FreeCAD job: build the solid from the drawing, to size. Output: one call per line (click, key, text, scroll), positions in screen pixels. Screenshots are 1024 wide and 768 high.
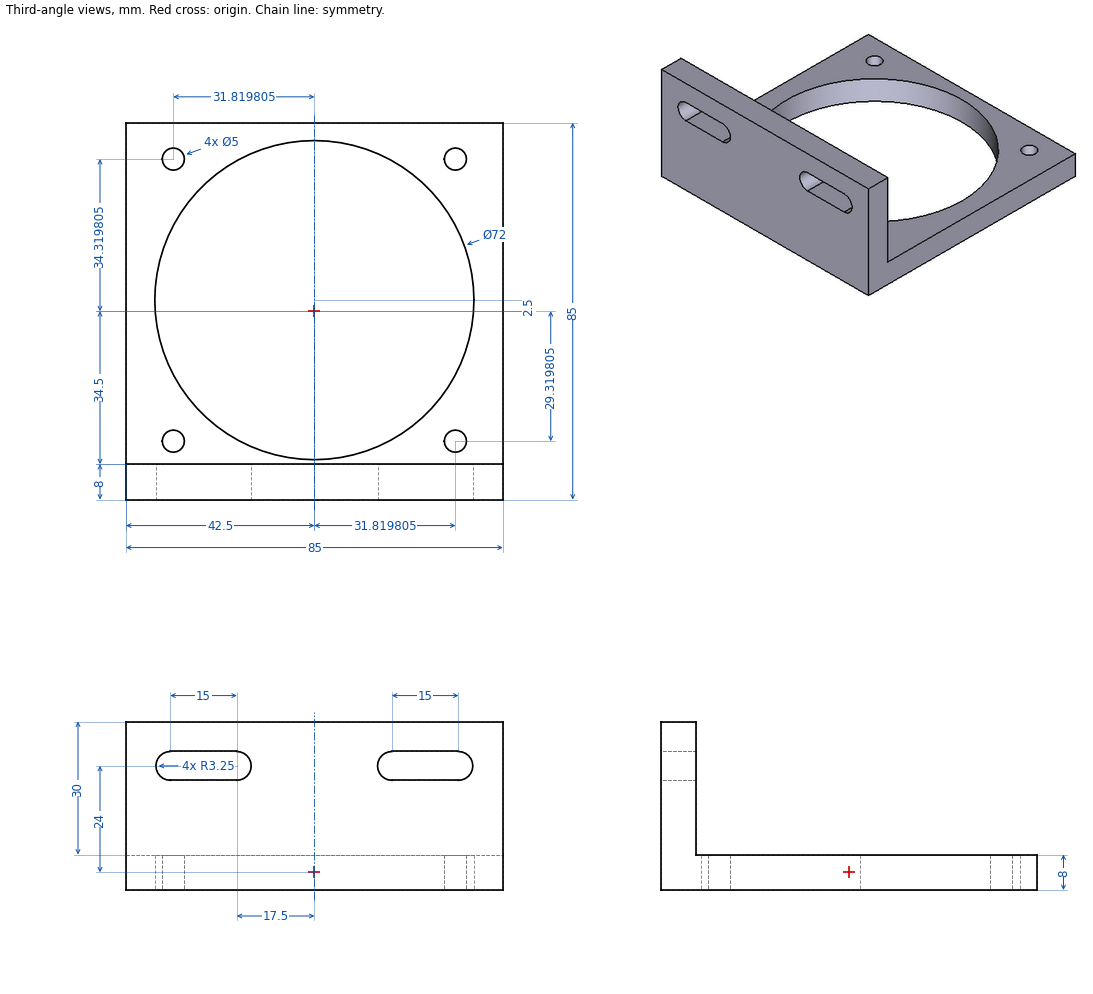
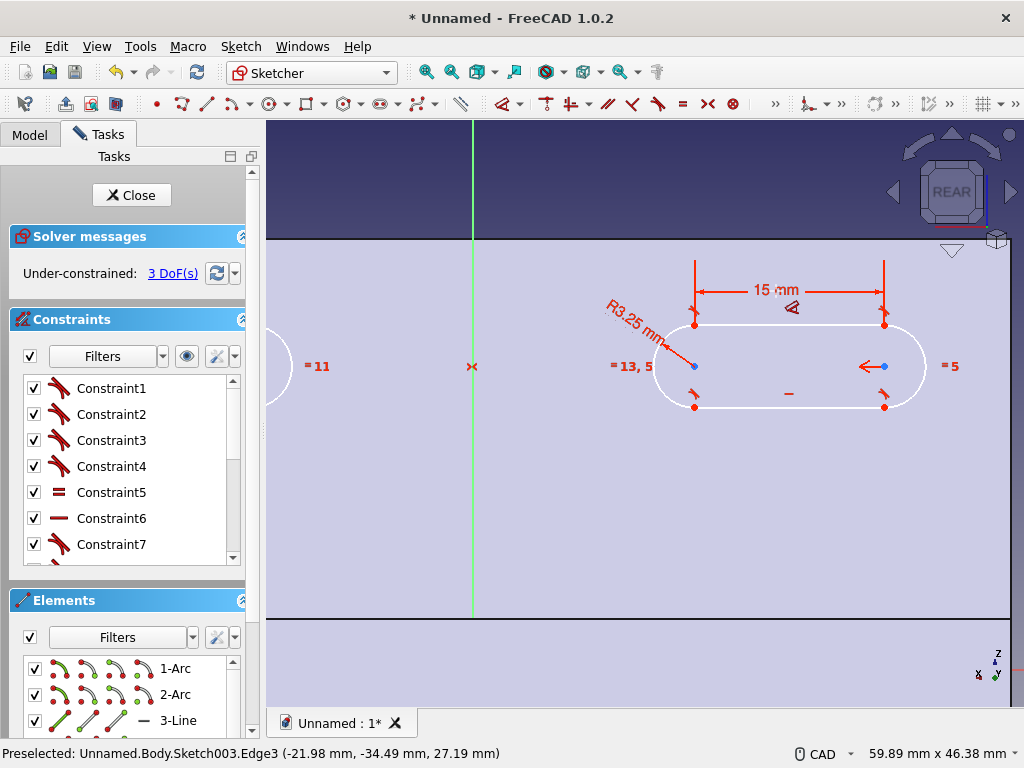
scroll(661, 345, down, 4)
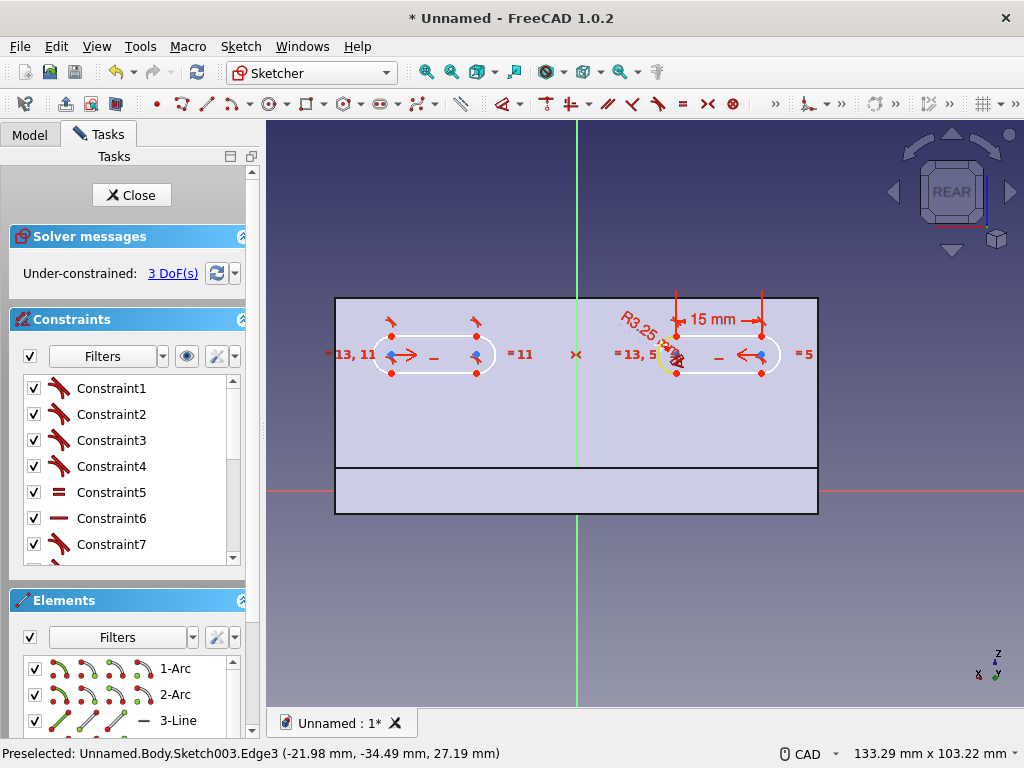
click(417, 336)
click(434, 302)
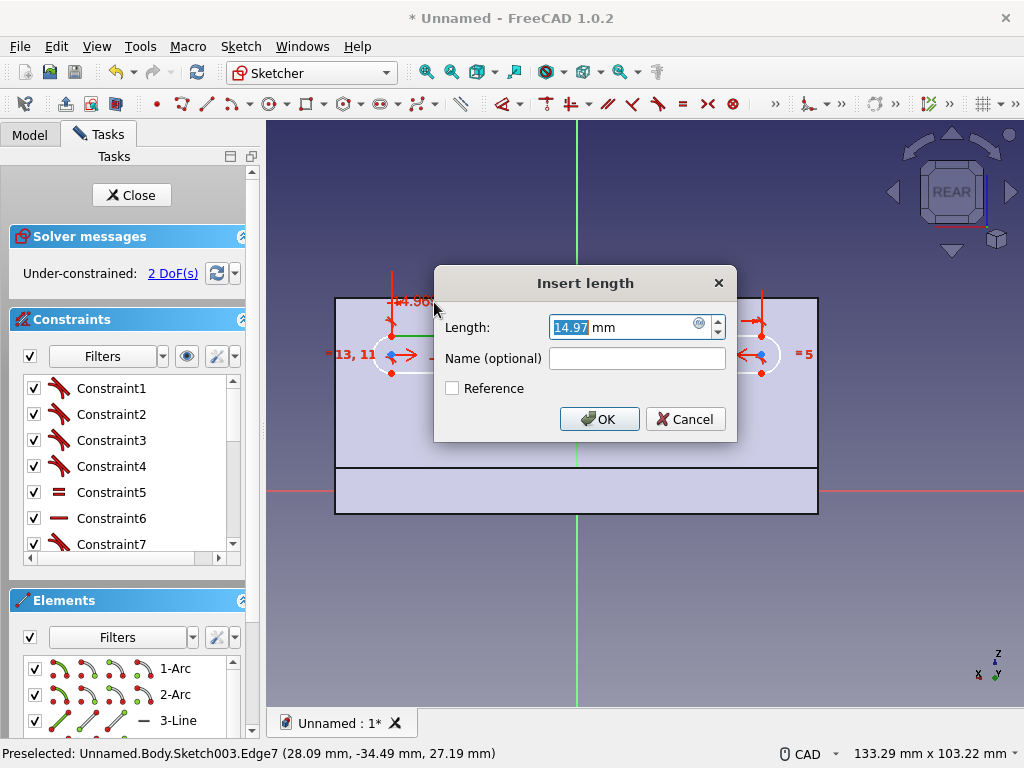
text(15)
key(Return)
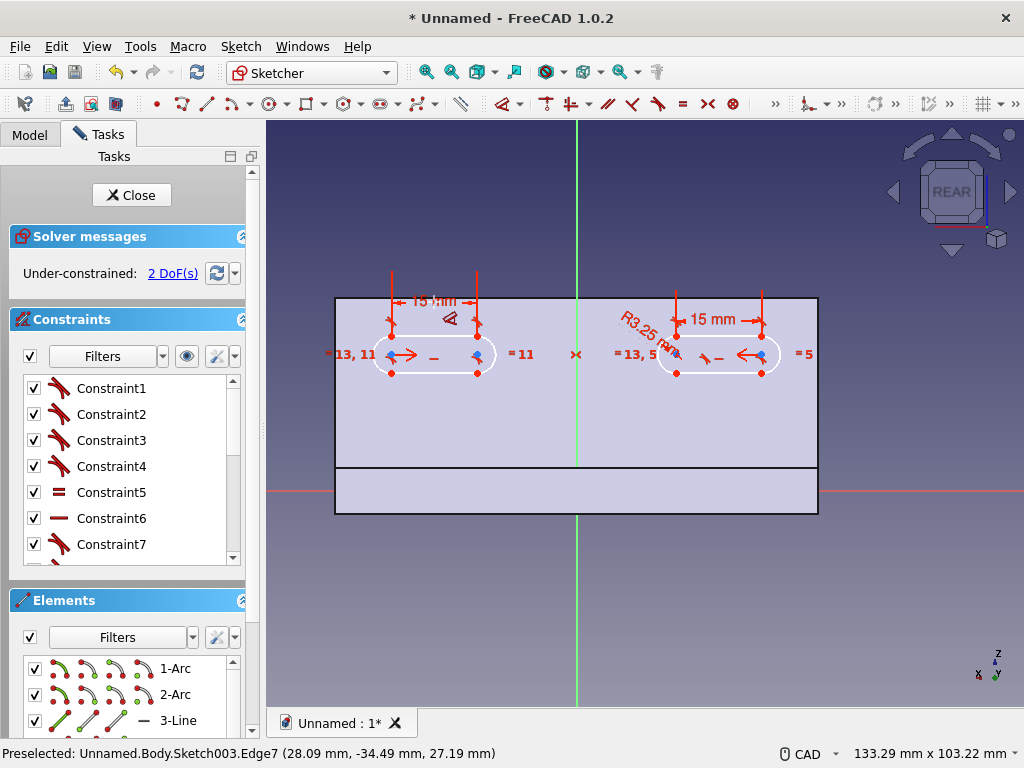
click(676, 355)
click(710, 423)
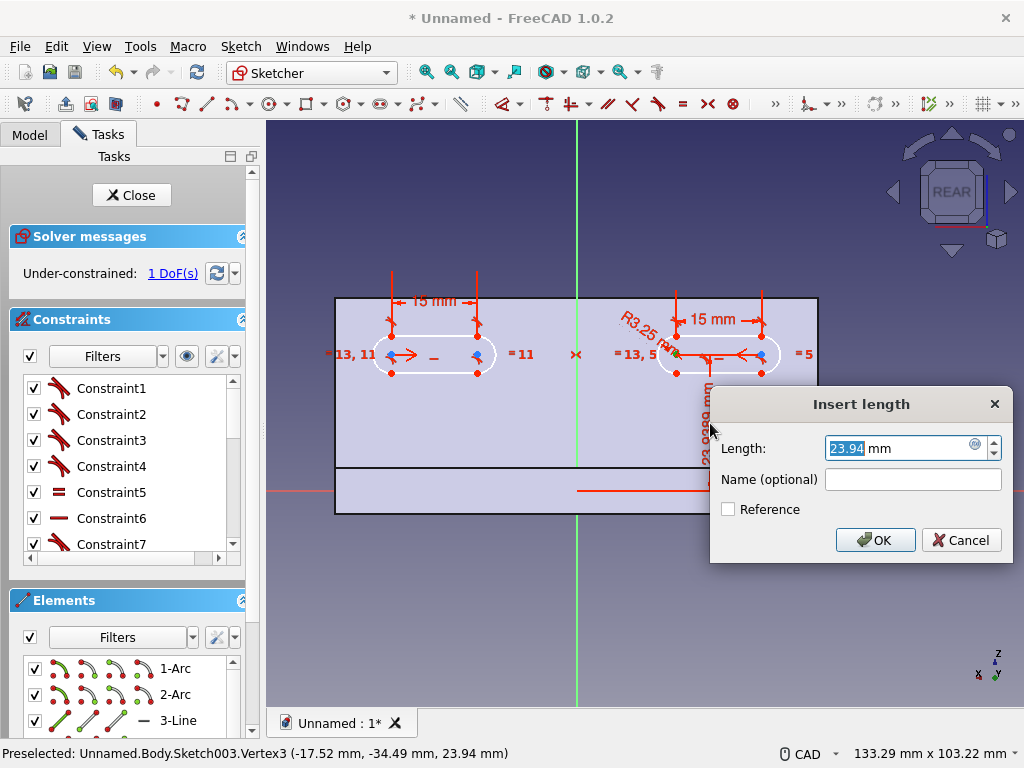
text(24)
key(Return)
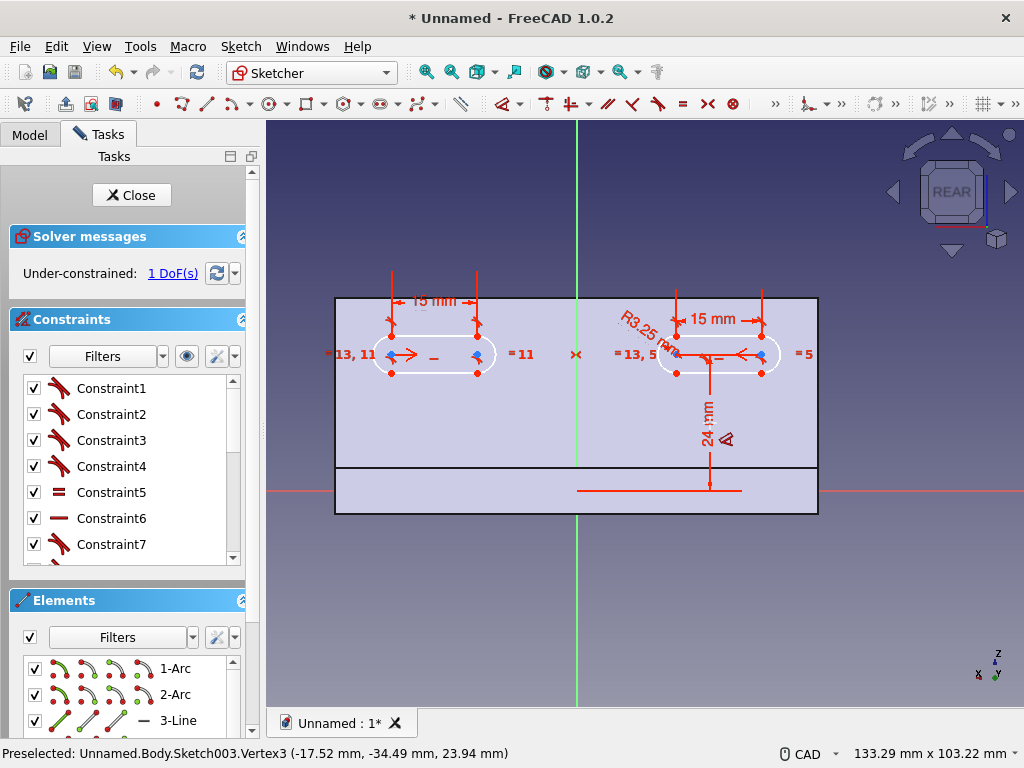
click(676, 336)
click(627, 525)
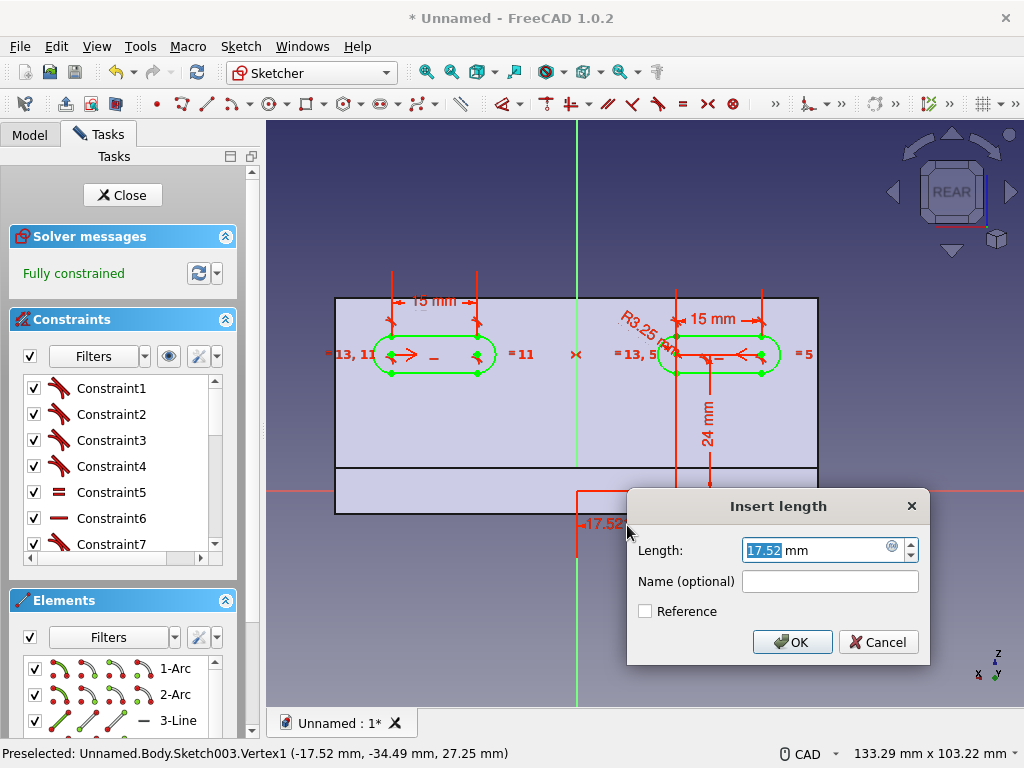
text(17.5)
key(Return)
key(Escape)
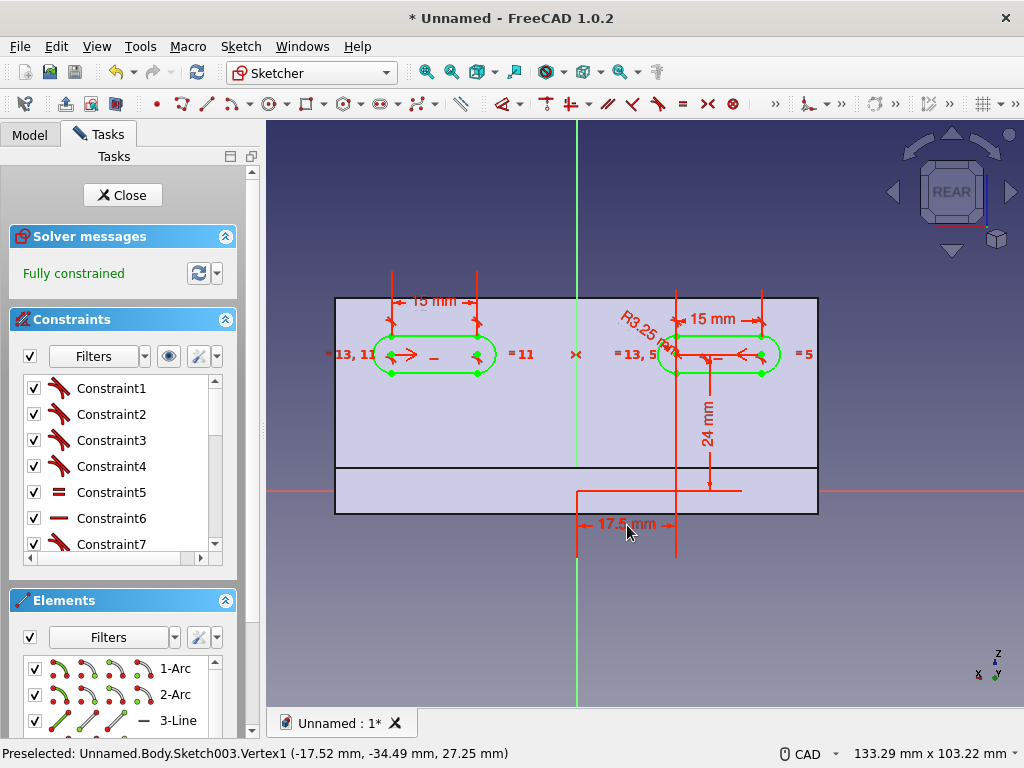
click(123, 195)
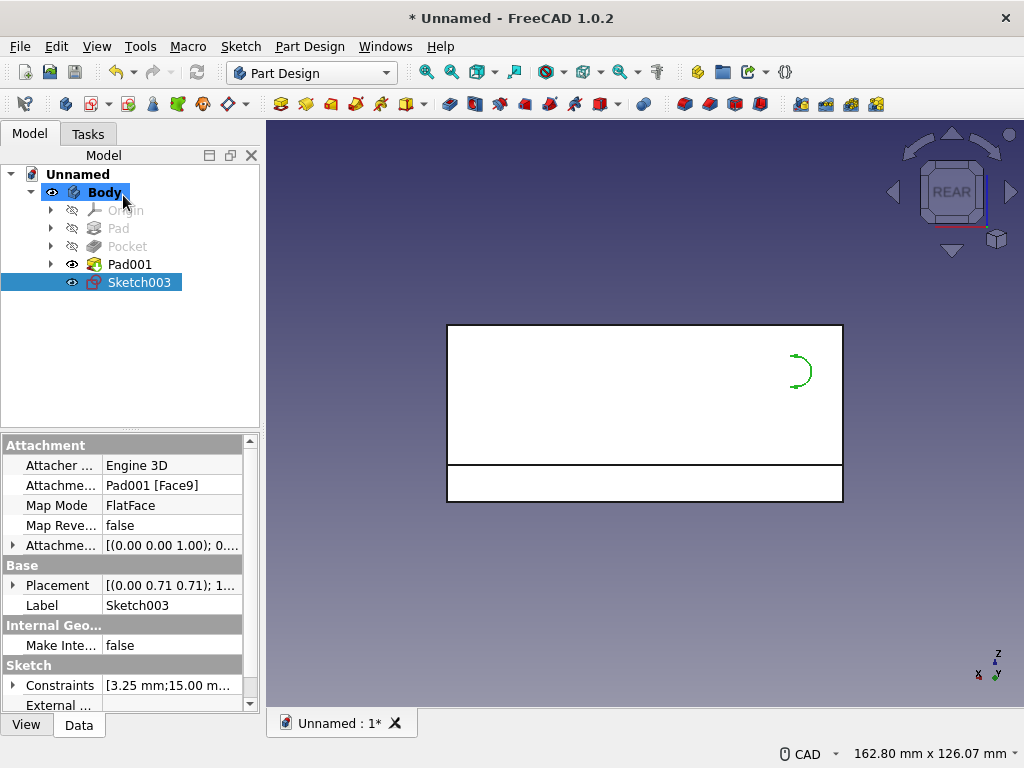
click(450, 104)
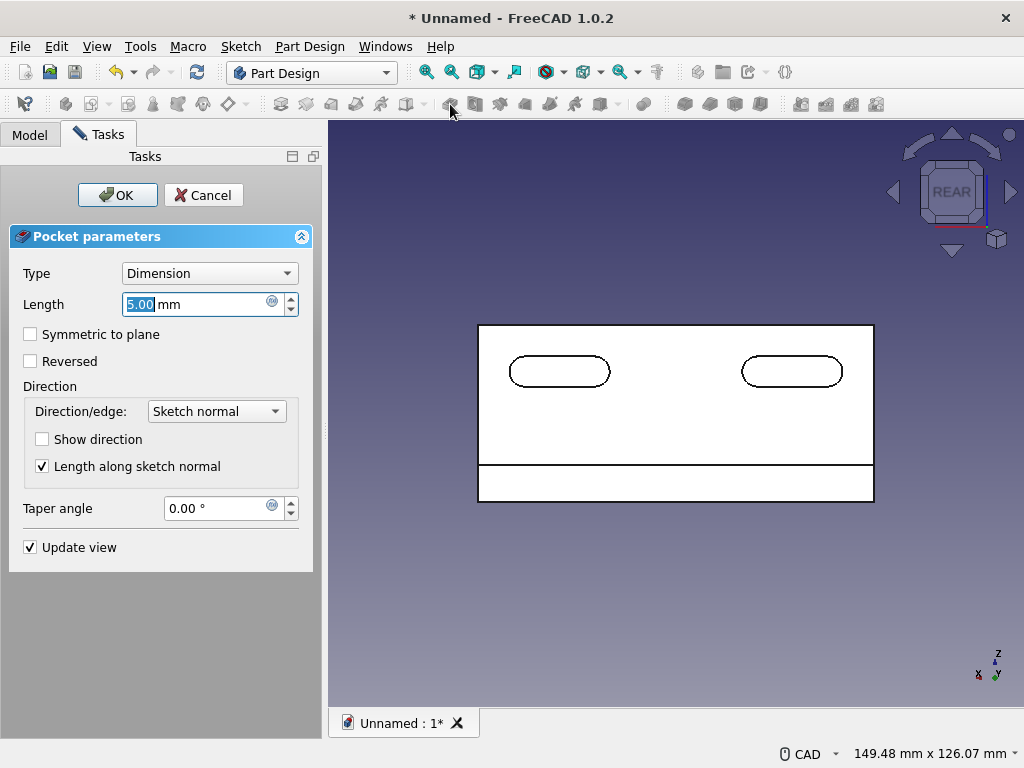
click(210, 274)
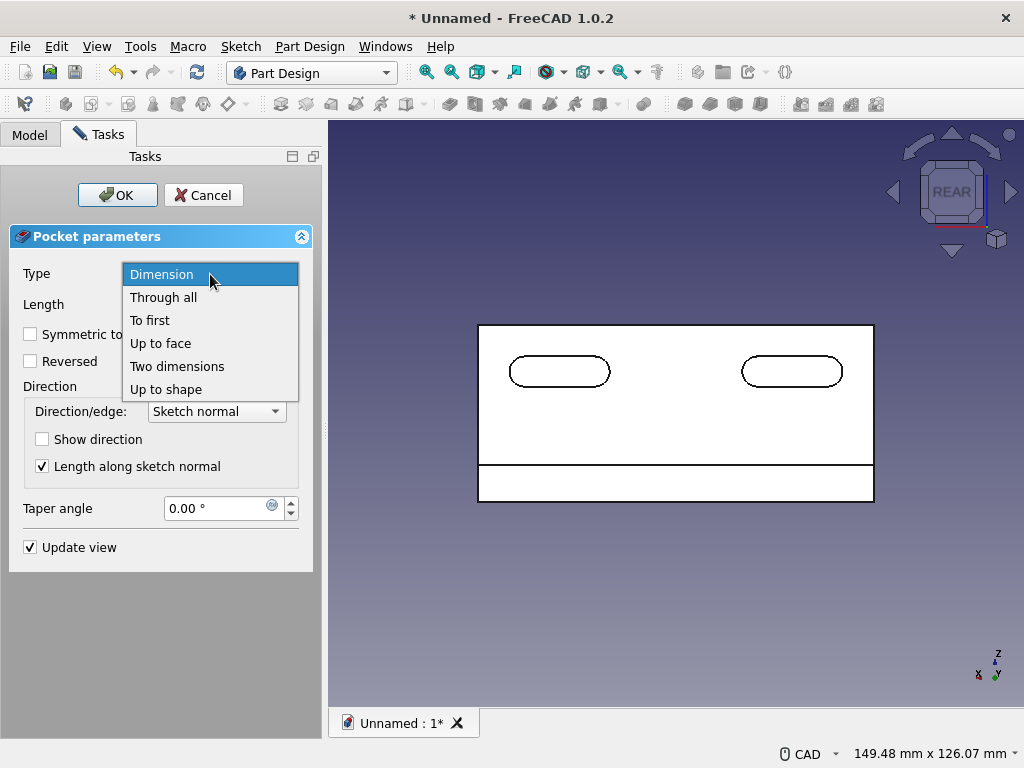
click(208, 298)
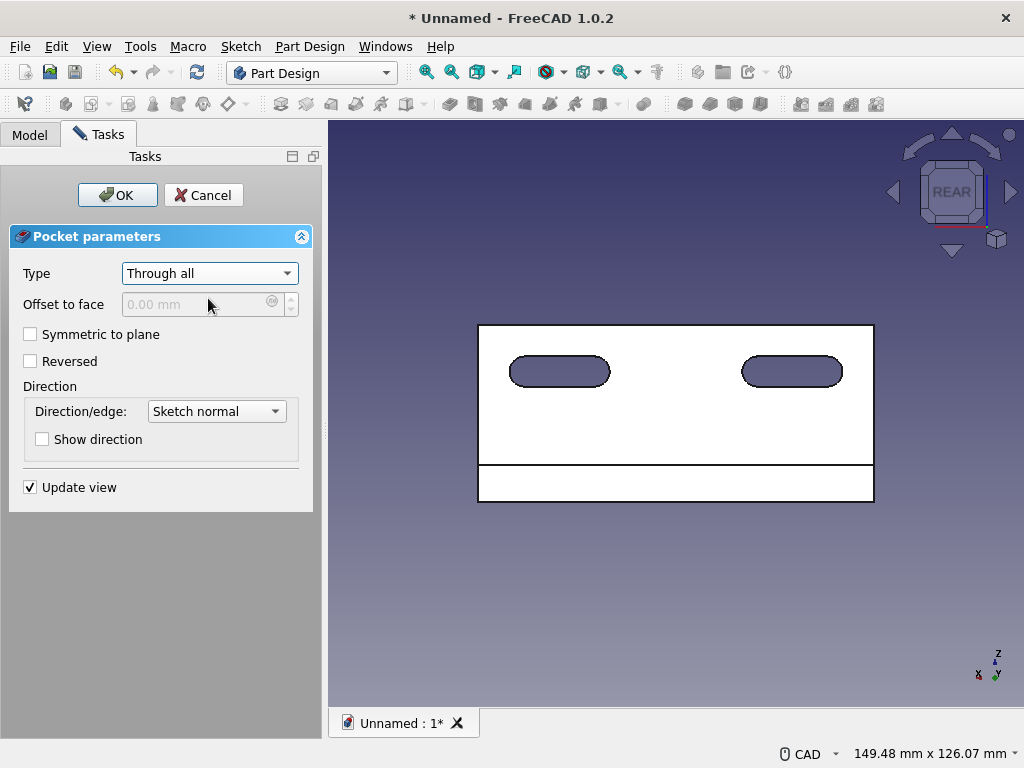
click(118, 195)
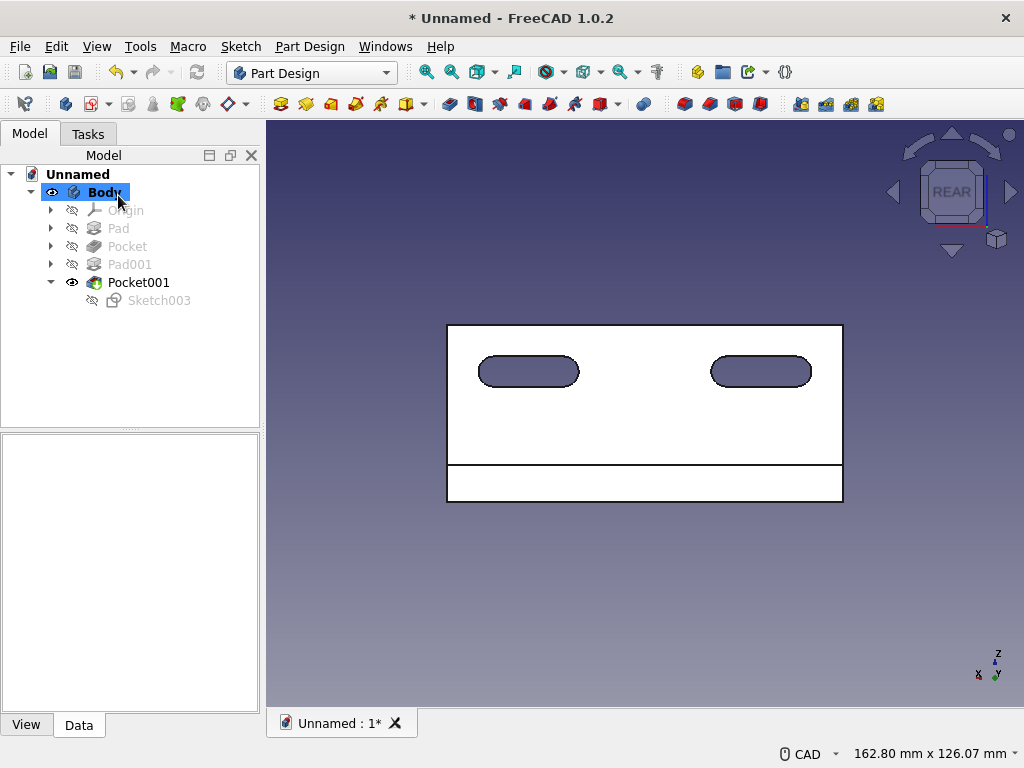
key(0)